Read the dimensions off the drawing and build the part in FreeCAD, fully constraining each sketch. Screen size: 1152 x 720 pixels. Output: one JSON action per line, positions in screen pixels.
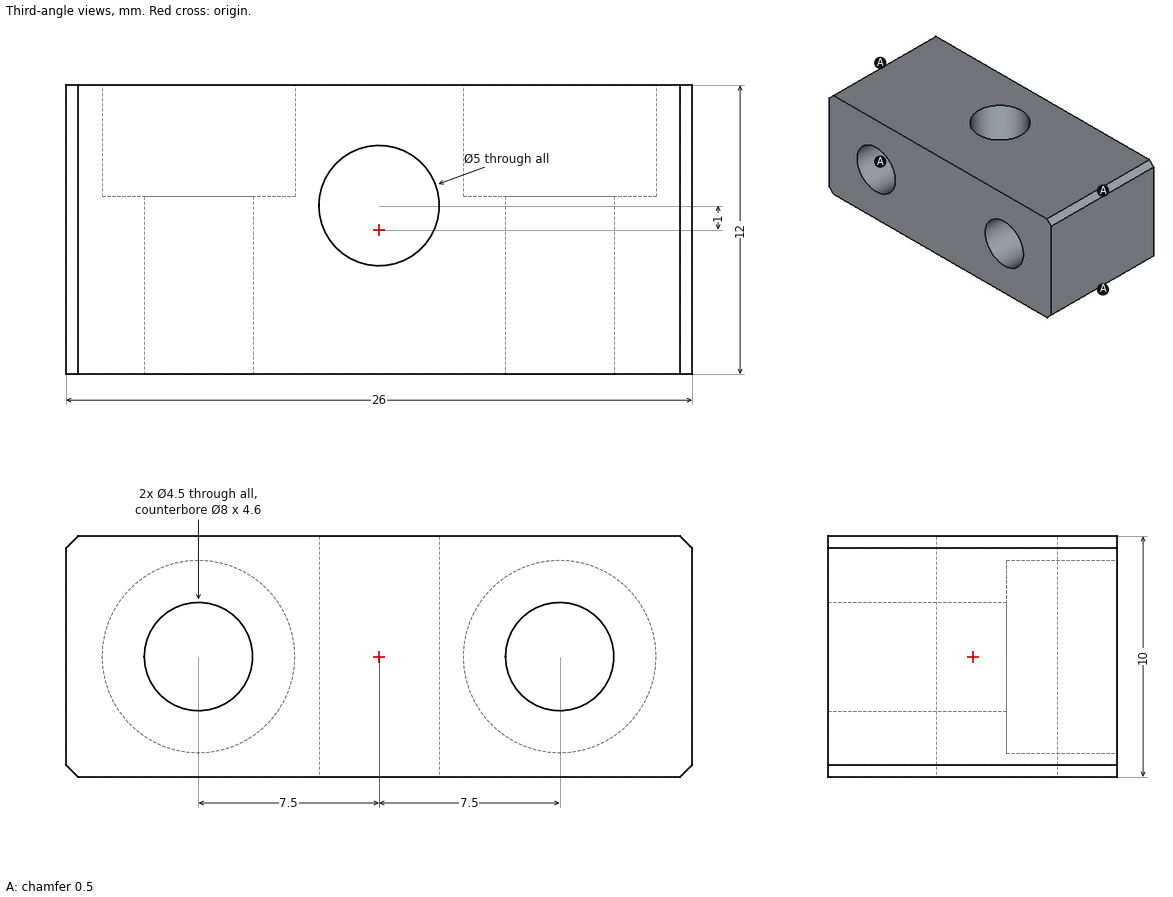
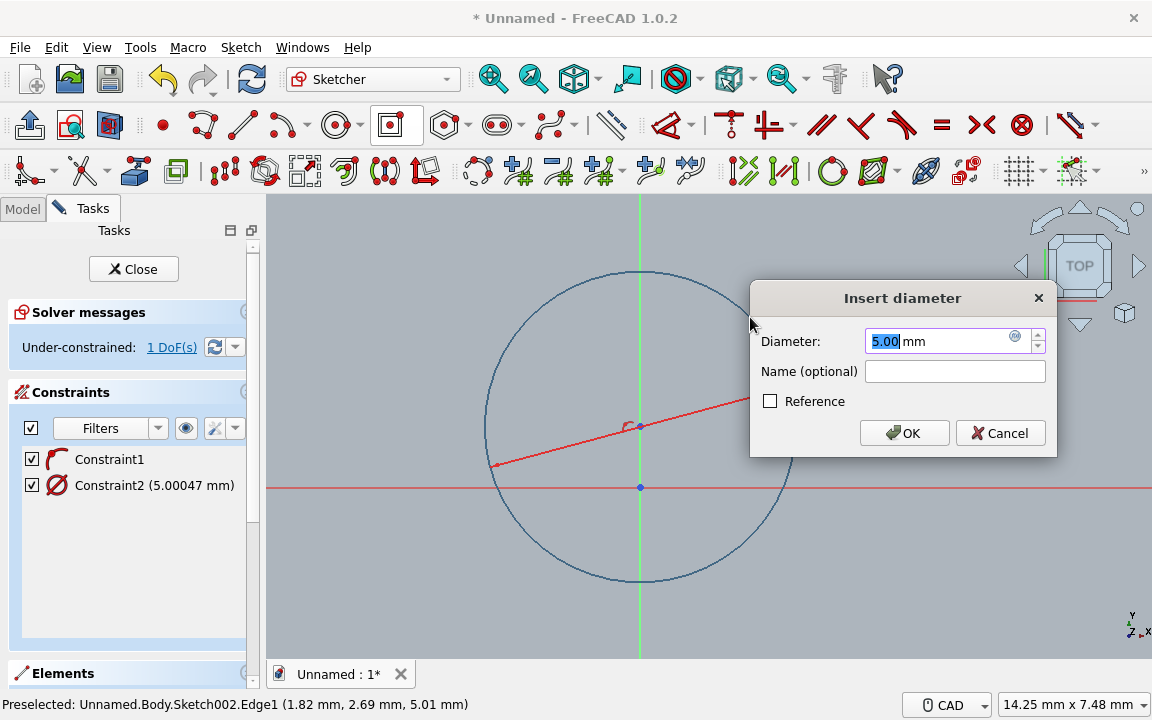
{"action": "type", "text": "5"}
{"action": "key", "text": "Return"}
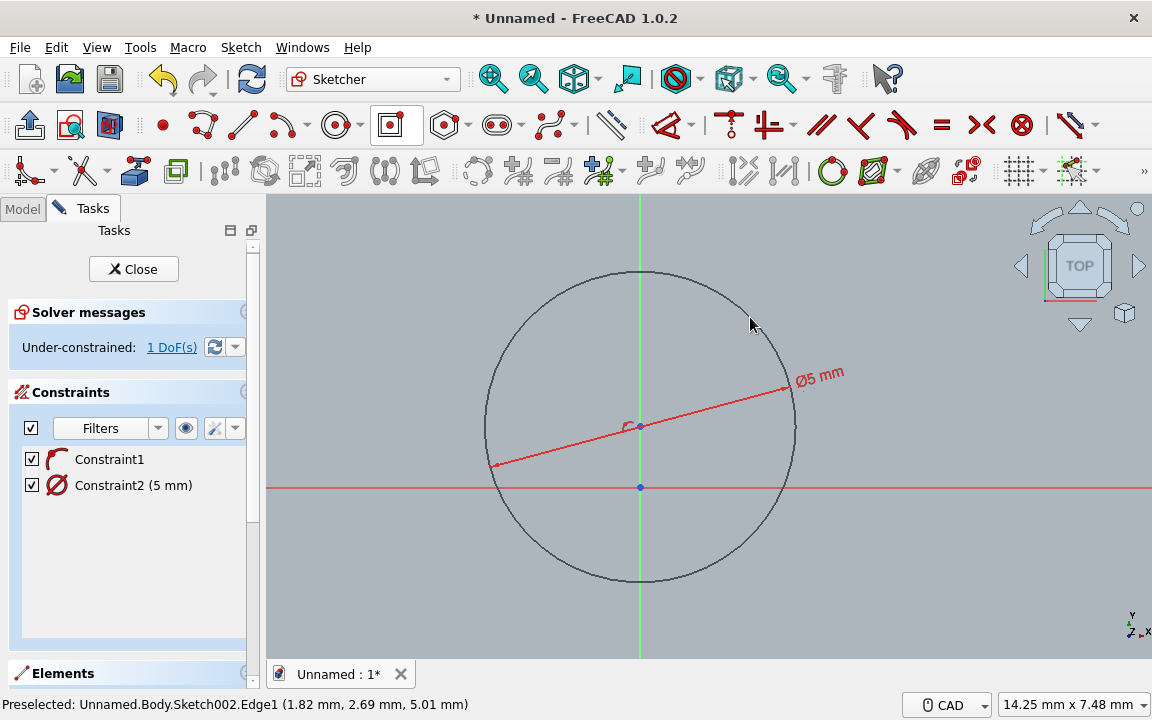
{"action": "left_click", "coordinate": [640, 427]}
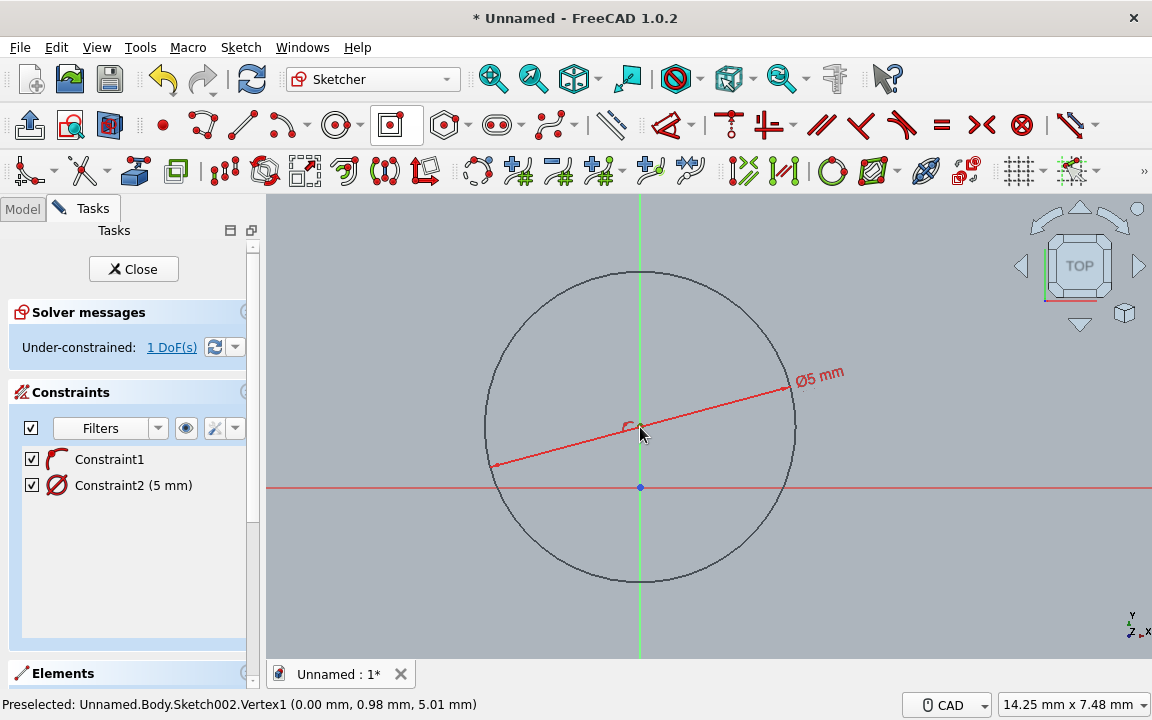
{"action": "key", "text": "i"}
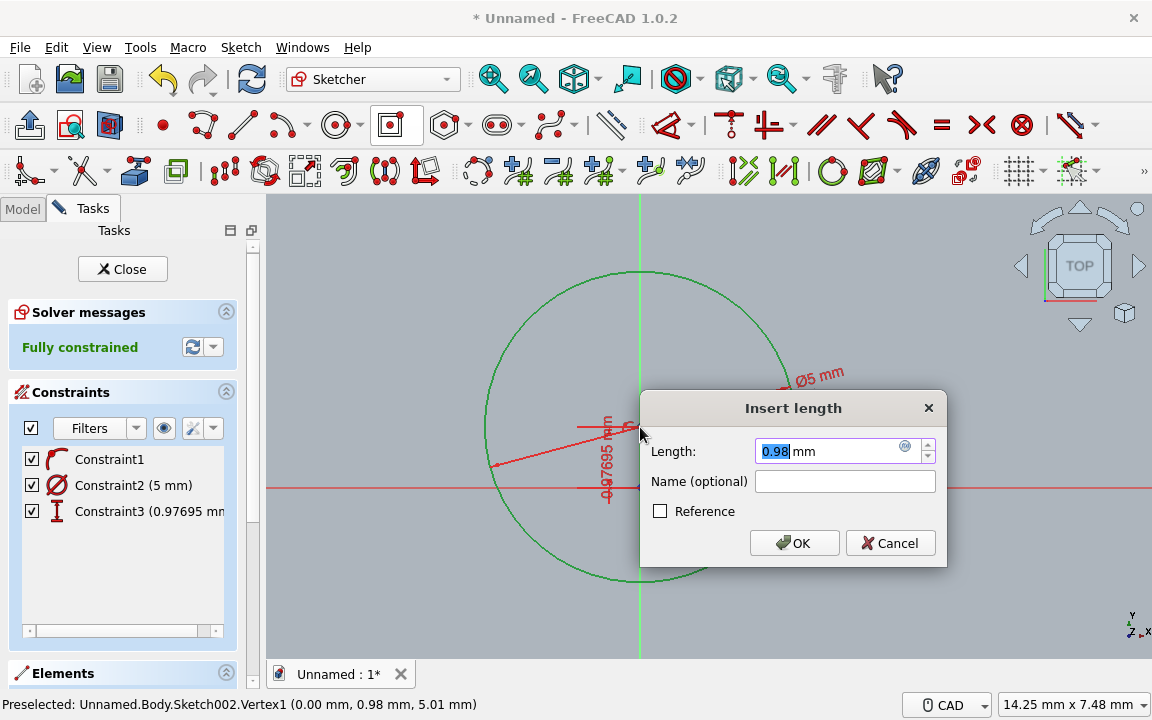
{"action": "type", "text": "1"}
{"action": "key", "text": "Return"}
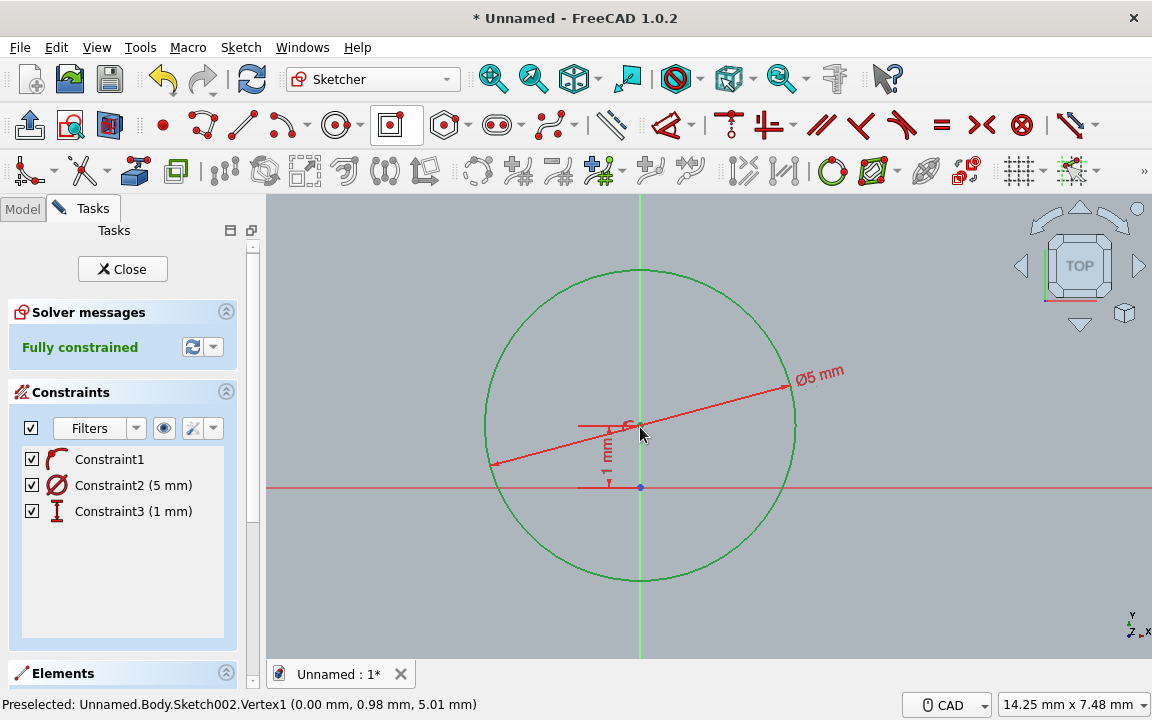
{"action": "left_click", "coordinate": [123, 269]}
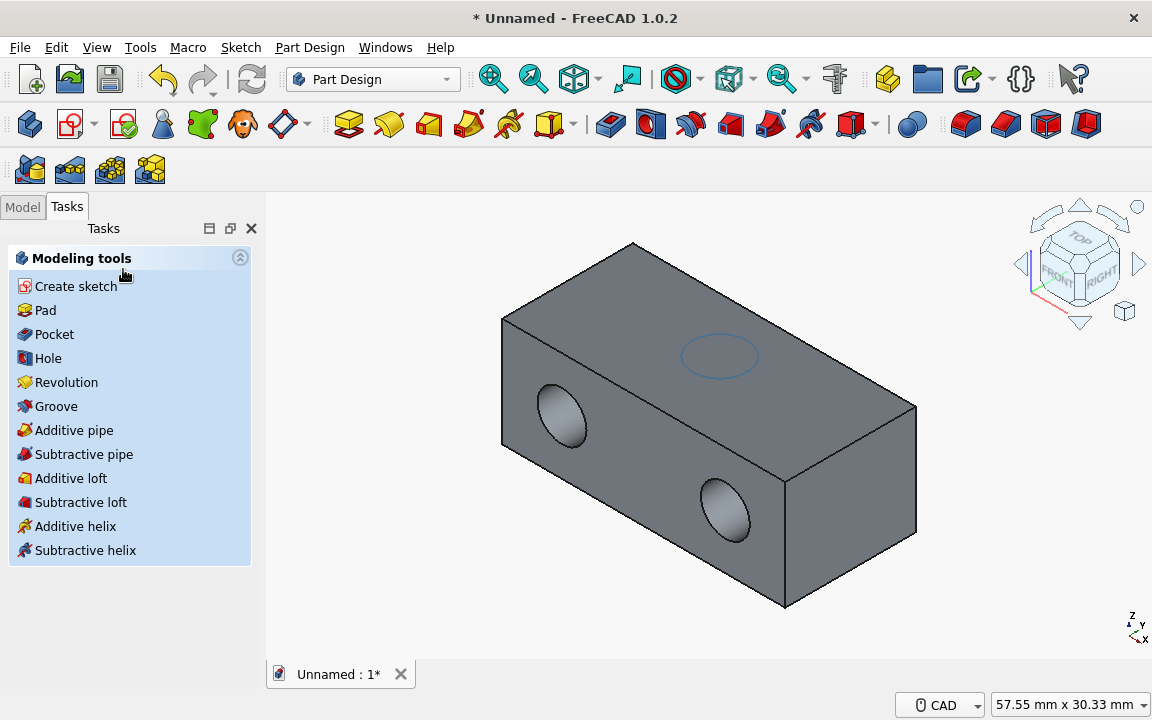
{"action": "left_click", "coordinate": [652, 124]}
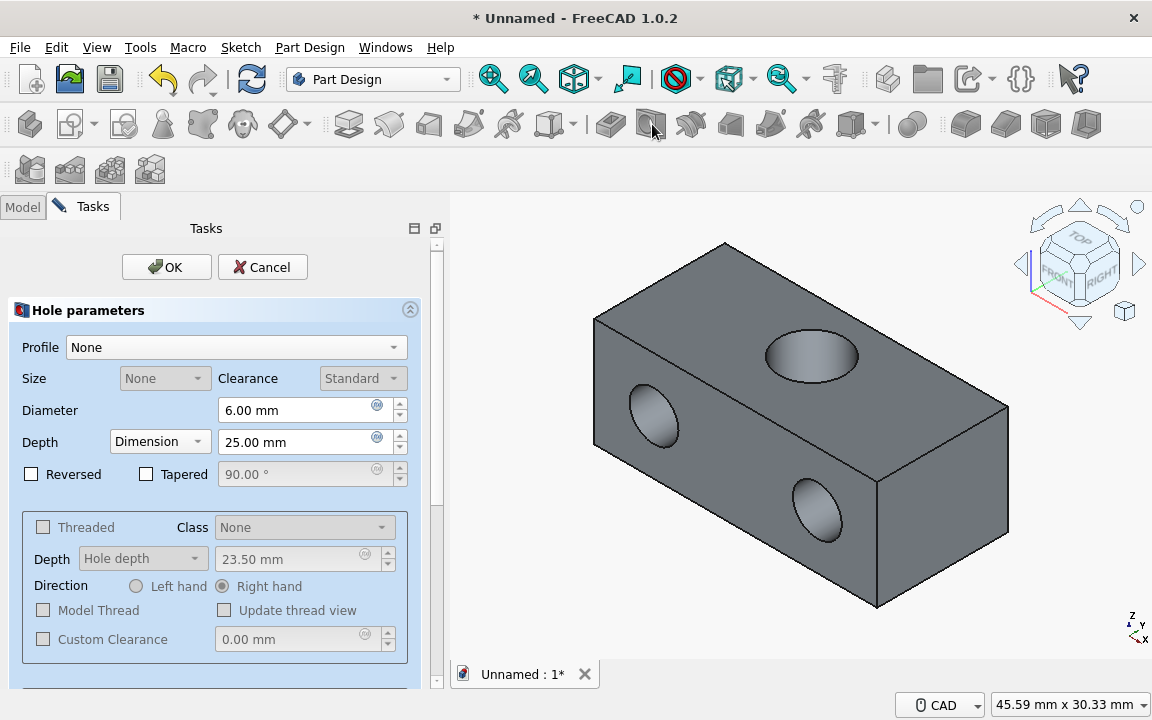
{"action": "triple_click", "coordinate": [305, 410]}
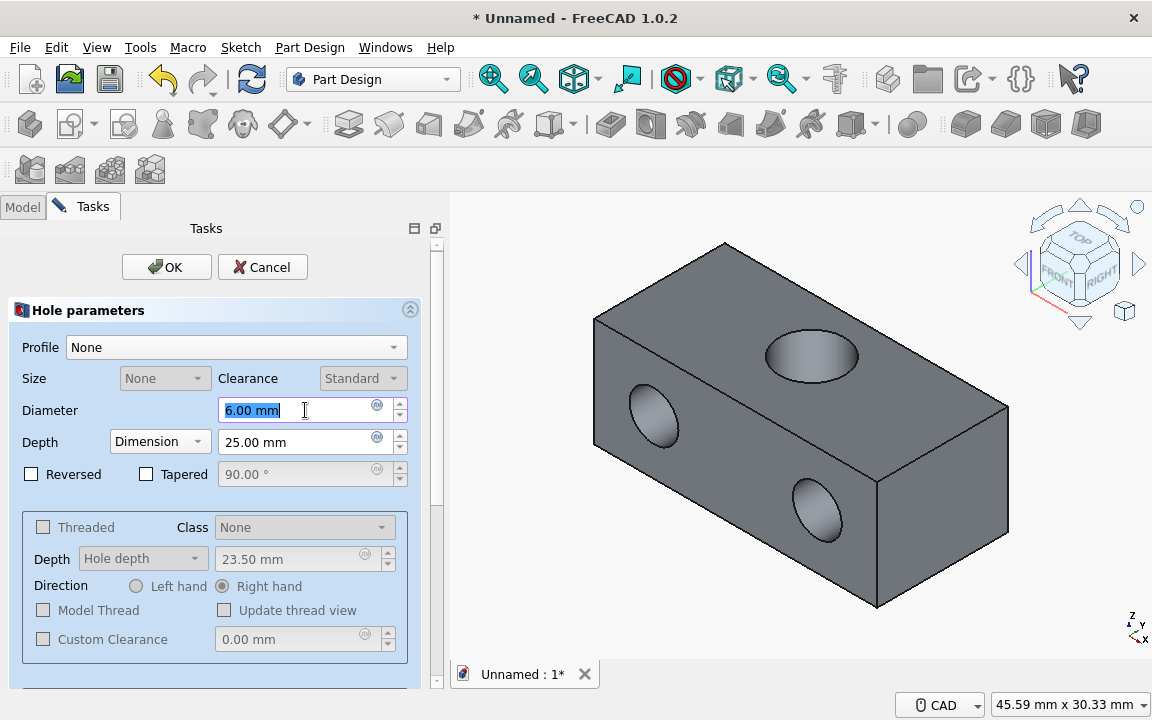
{"action": "type", "text": "5"}
{"action": "key", "text": "Tab"}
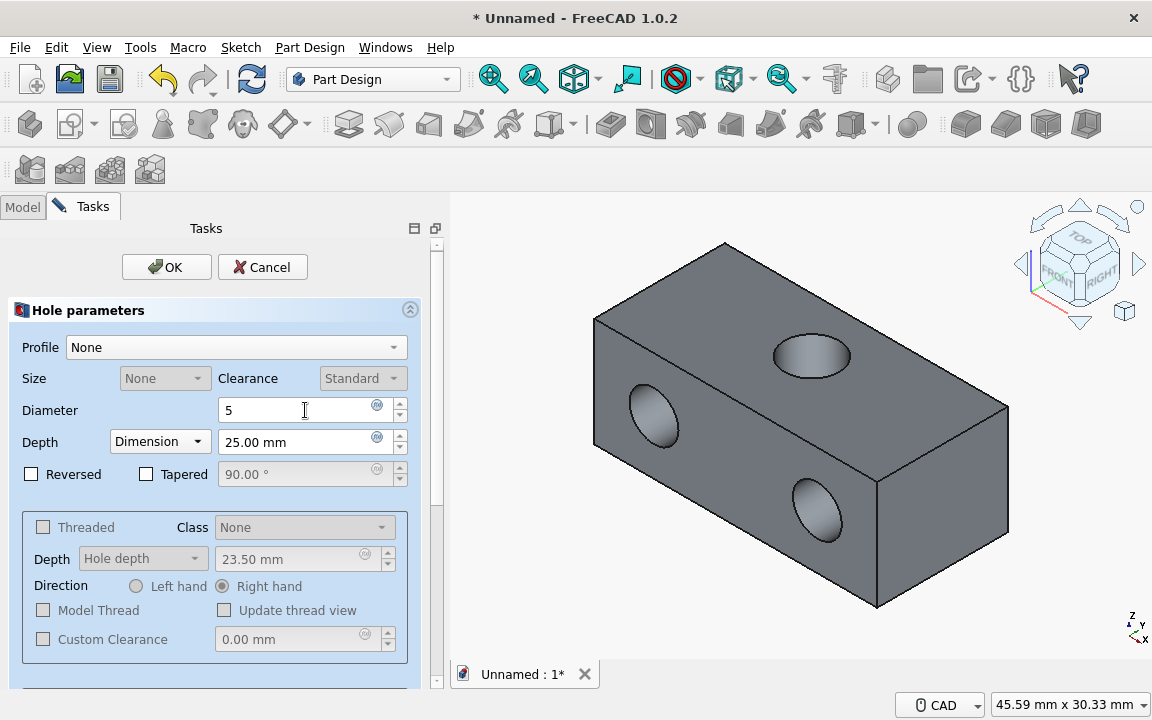
{"action": "left_click", "coordinate": [161, 442]}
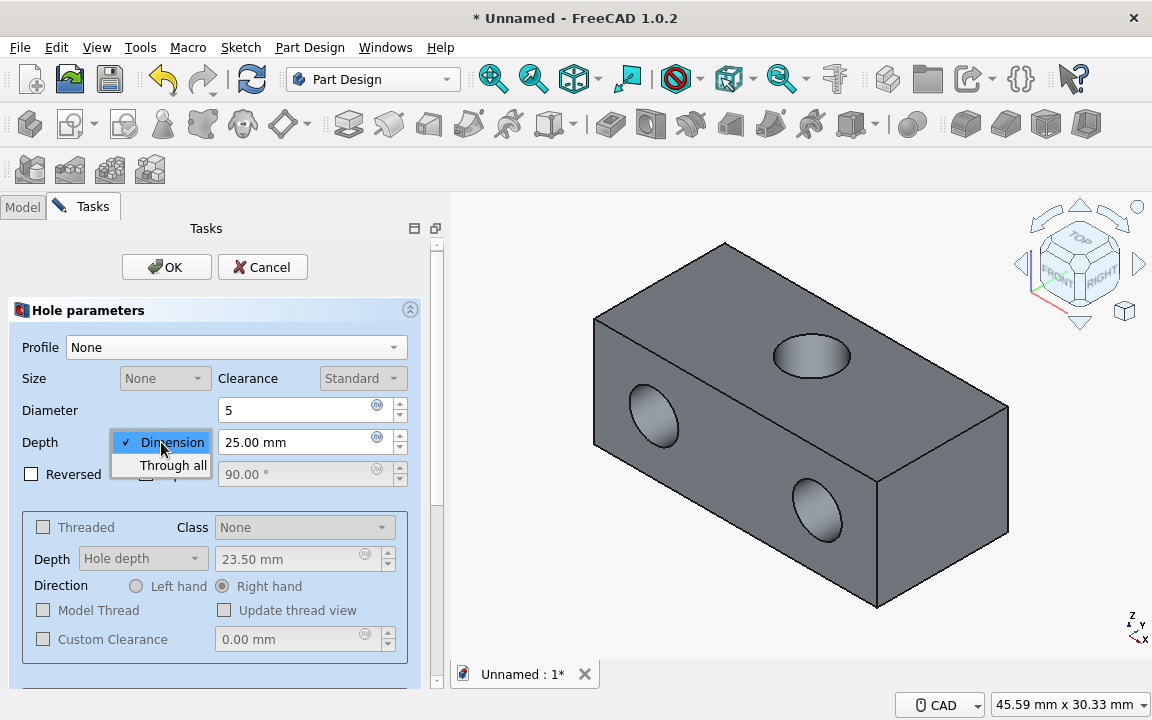
{"action": "left_click", "coordinate": [160, 466]}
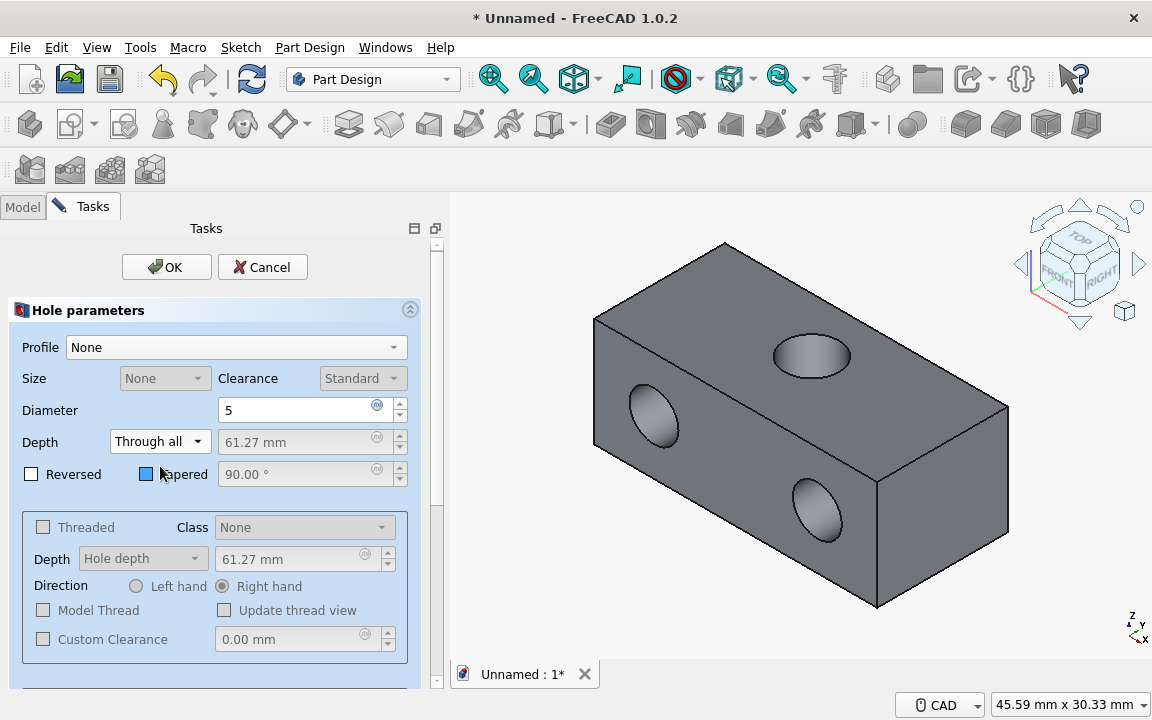
{"action": "left_click", "coordinate": [167, 267]}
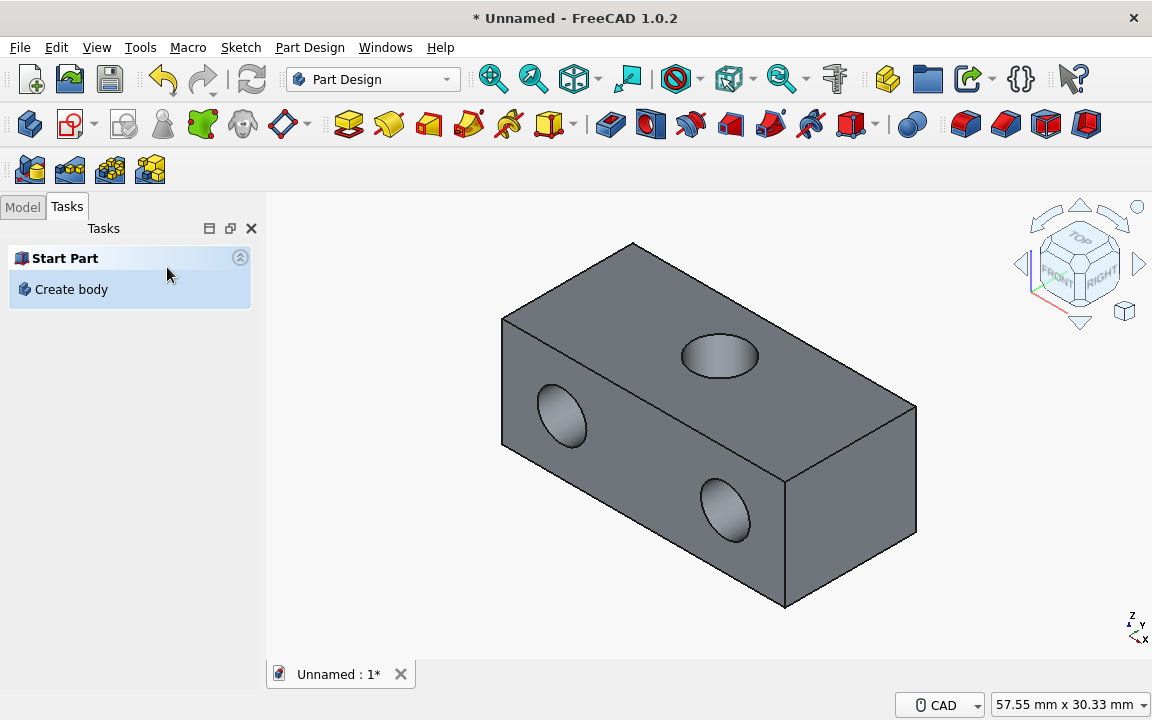
{"action": "left_click", "coordinate": [851, 443]}